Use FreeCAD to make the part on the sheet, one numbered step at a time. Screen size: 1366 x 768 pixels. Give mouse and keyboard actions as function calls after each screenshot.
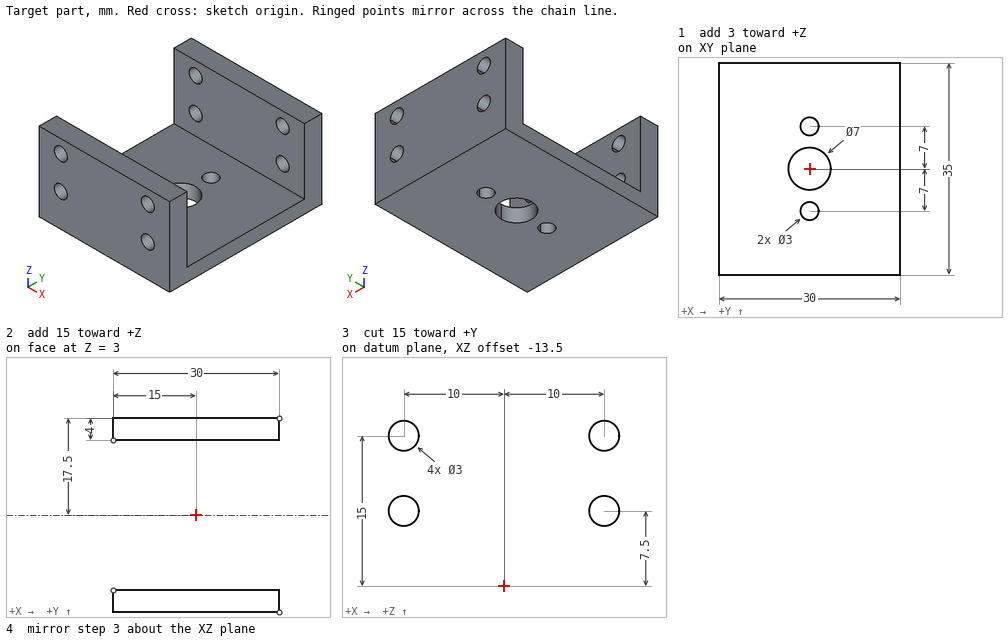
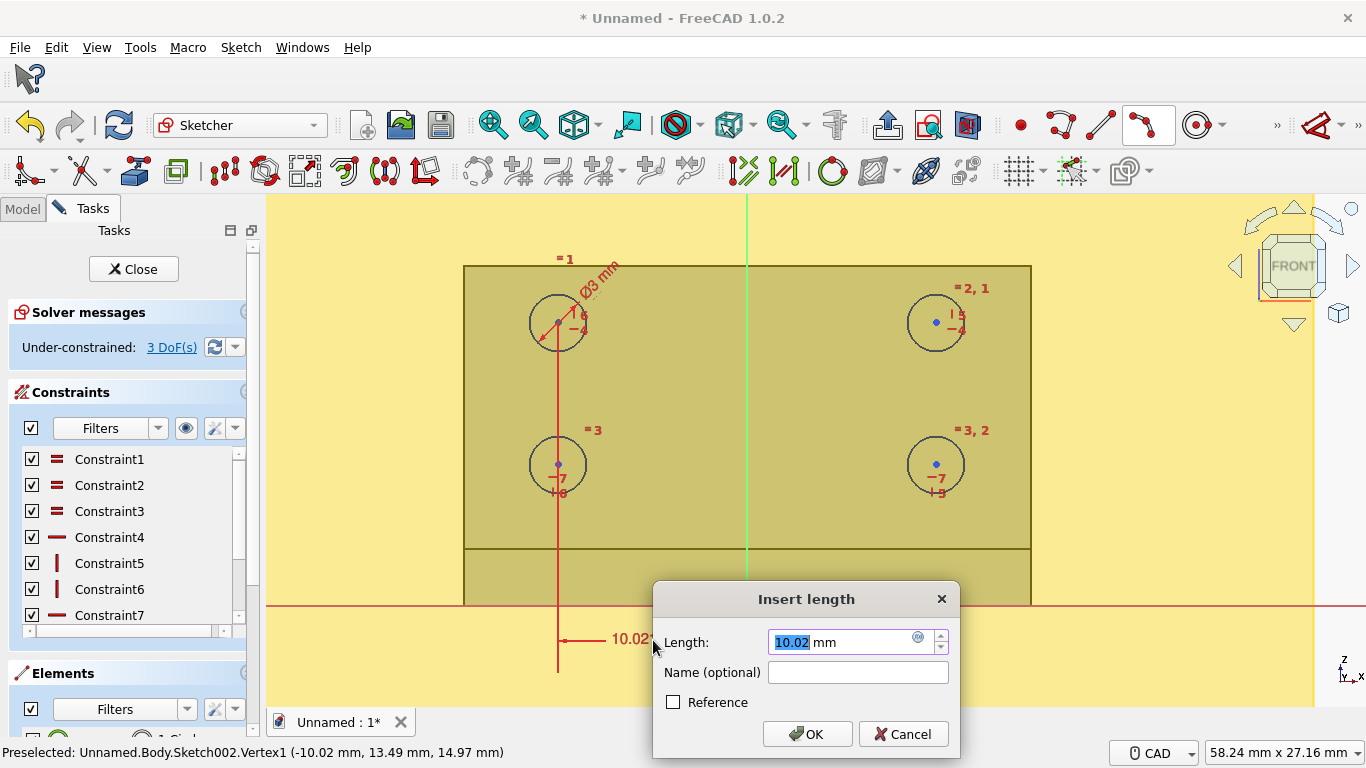
text(10)
key(Return)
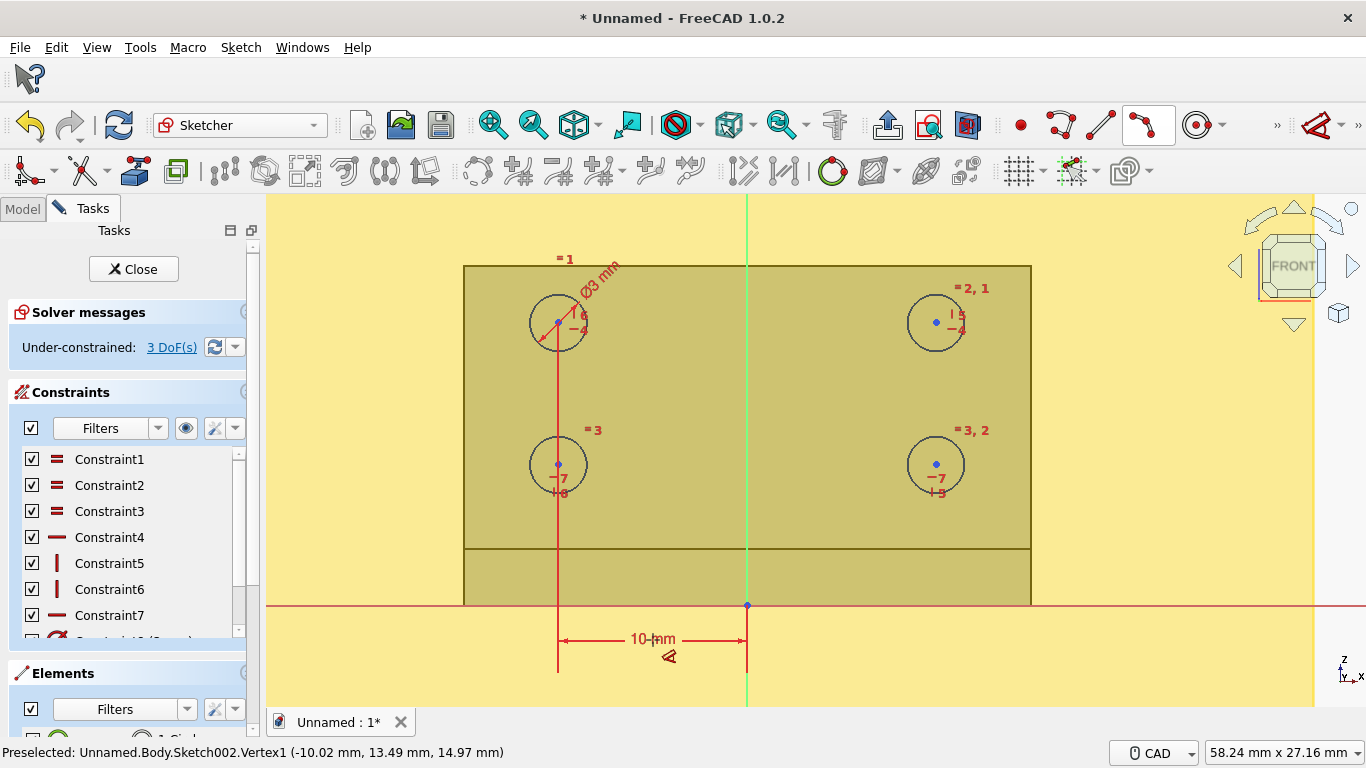
click(558, 323)
click(524, 399)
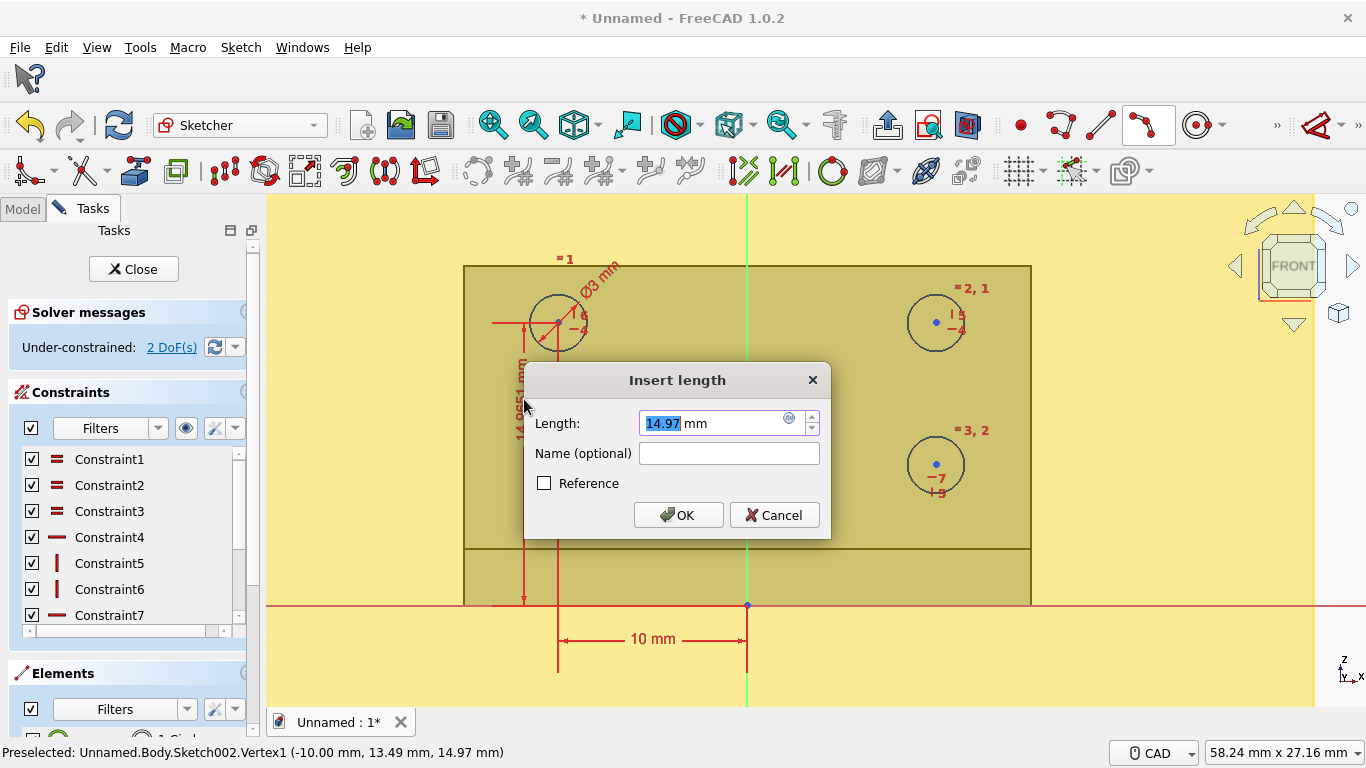
text(15)
key(Return)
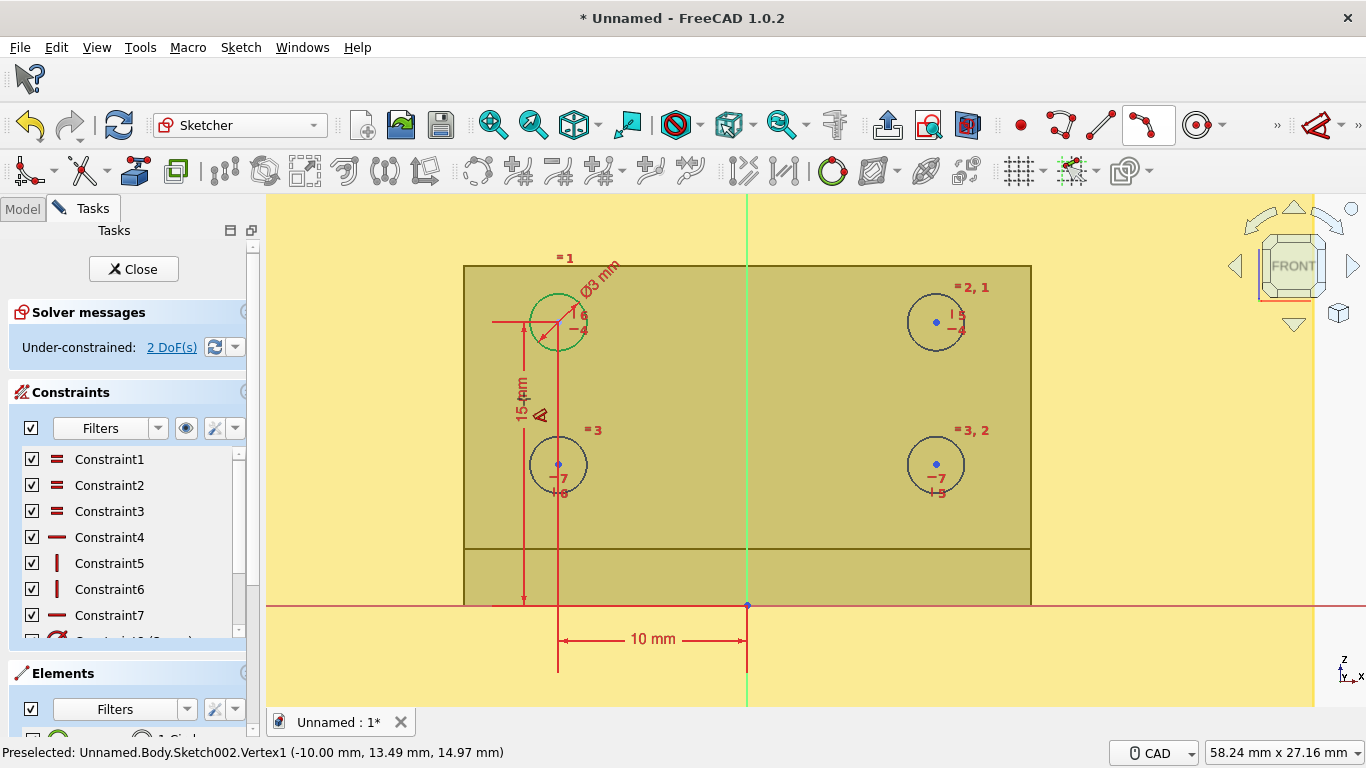
click(936, 322)
click(842, 640)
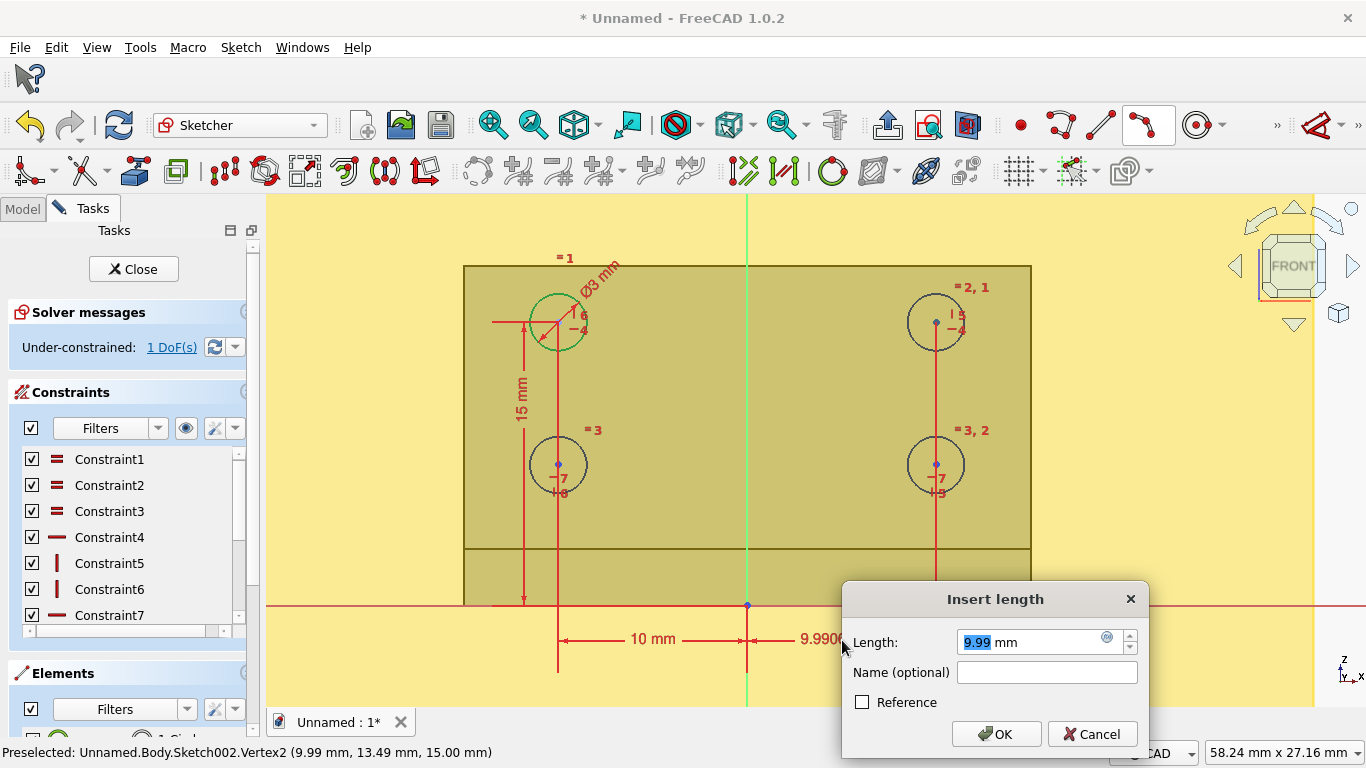
text(10)
key(Return)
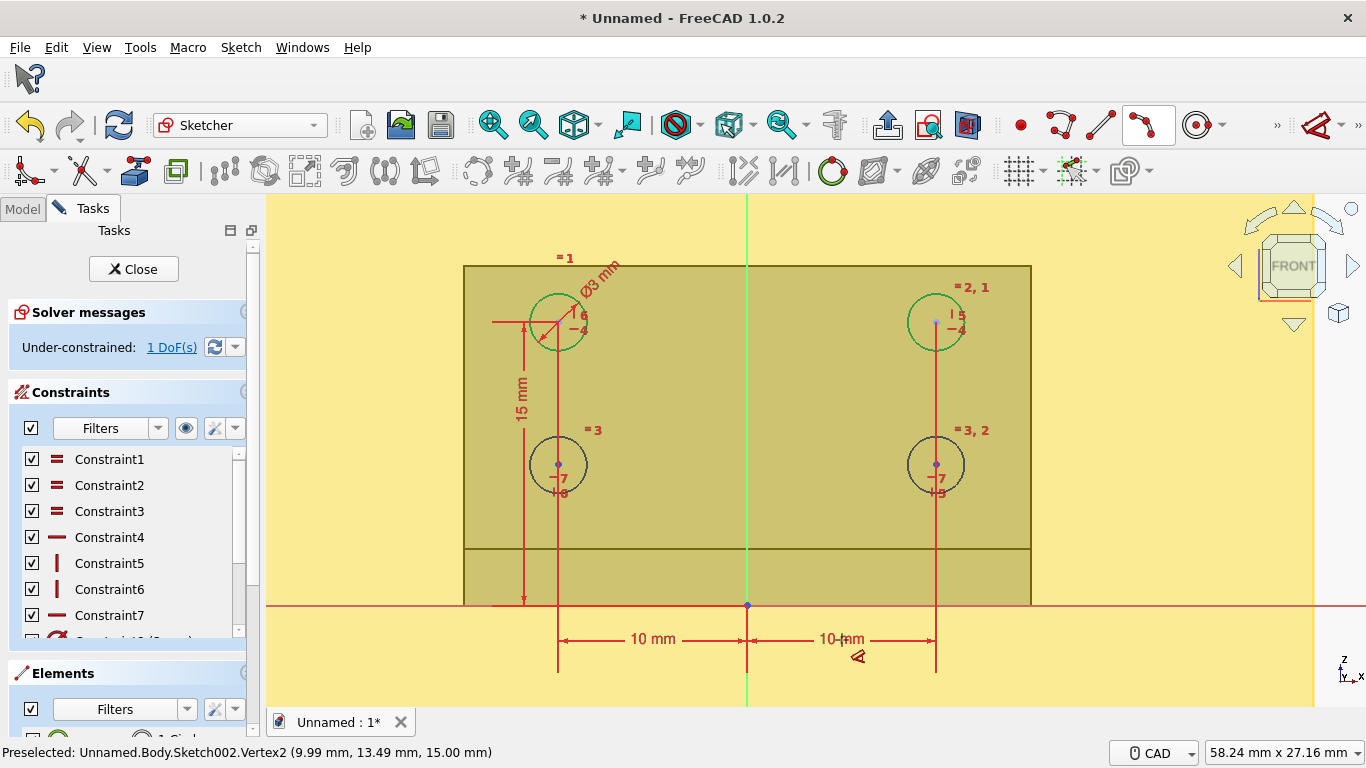
click(936, 465)
click(970, 535)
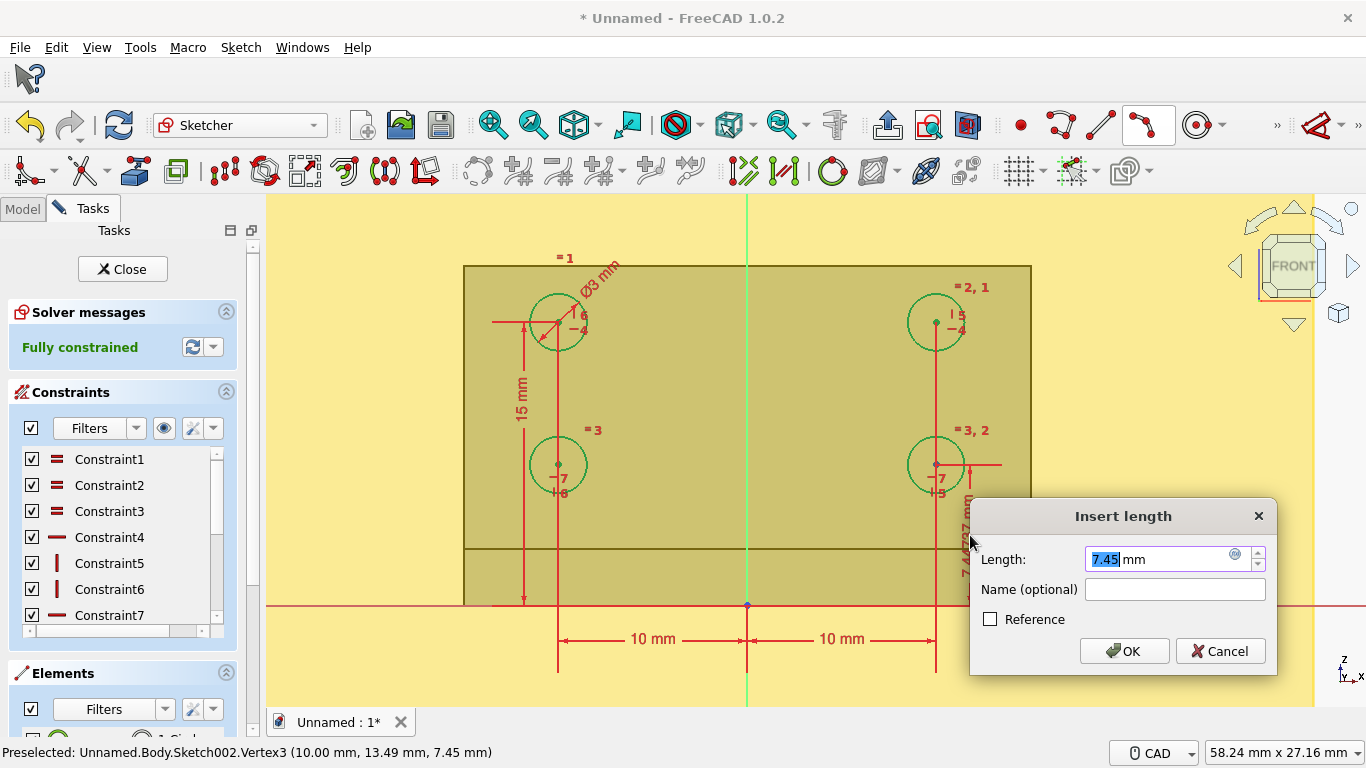
text(7.5)
key(Return)
key(Escape)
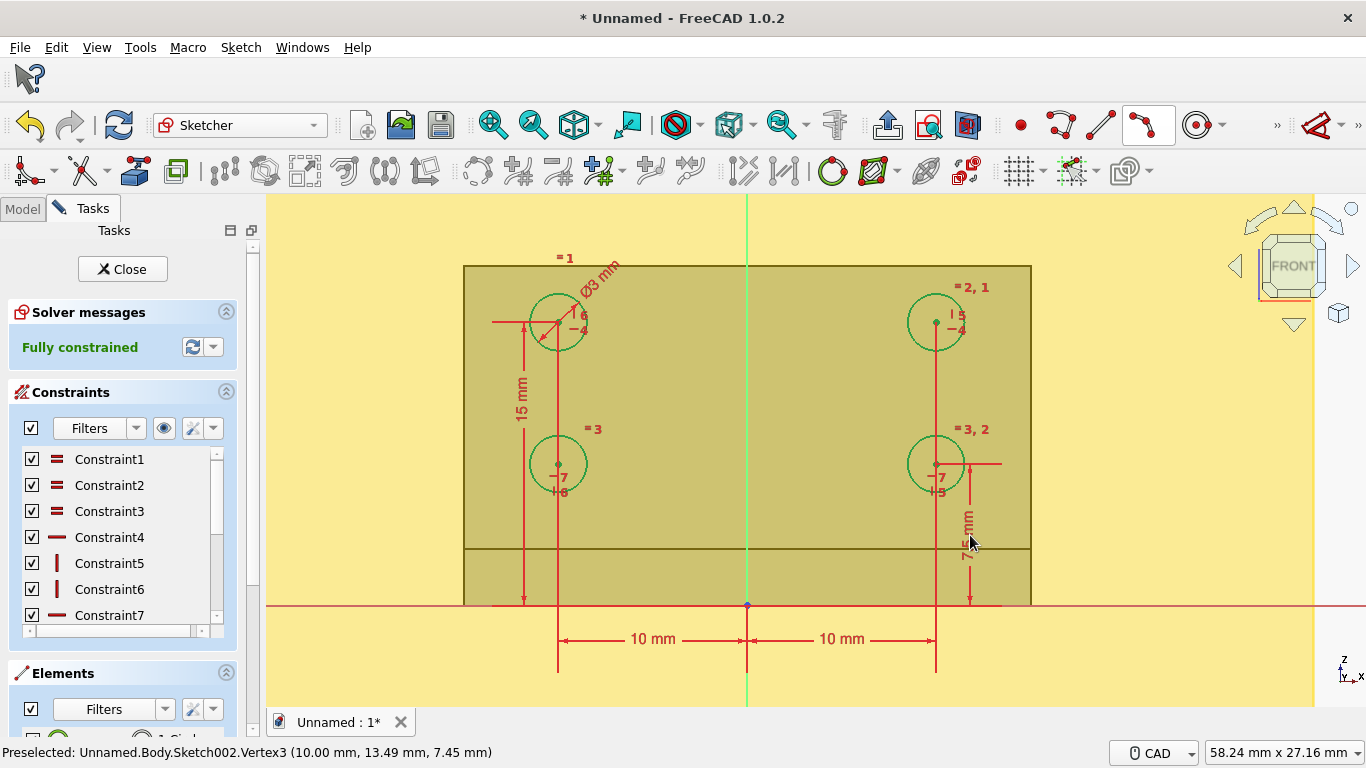
click(123, 269)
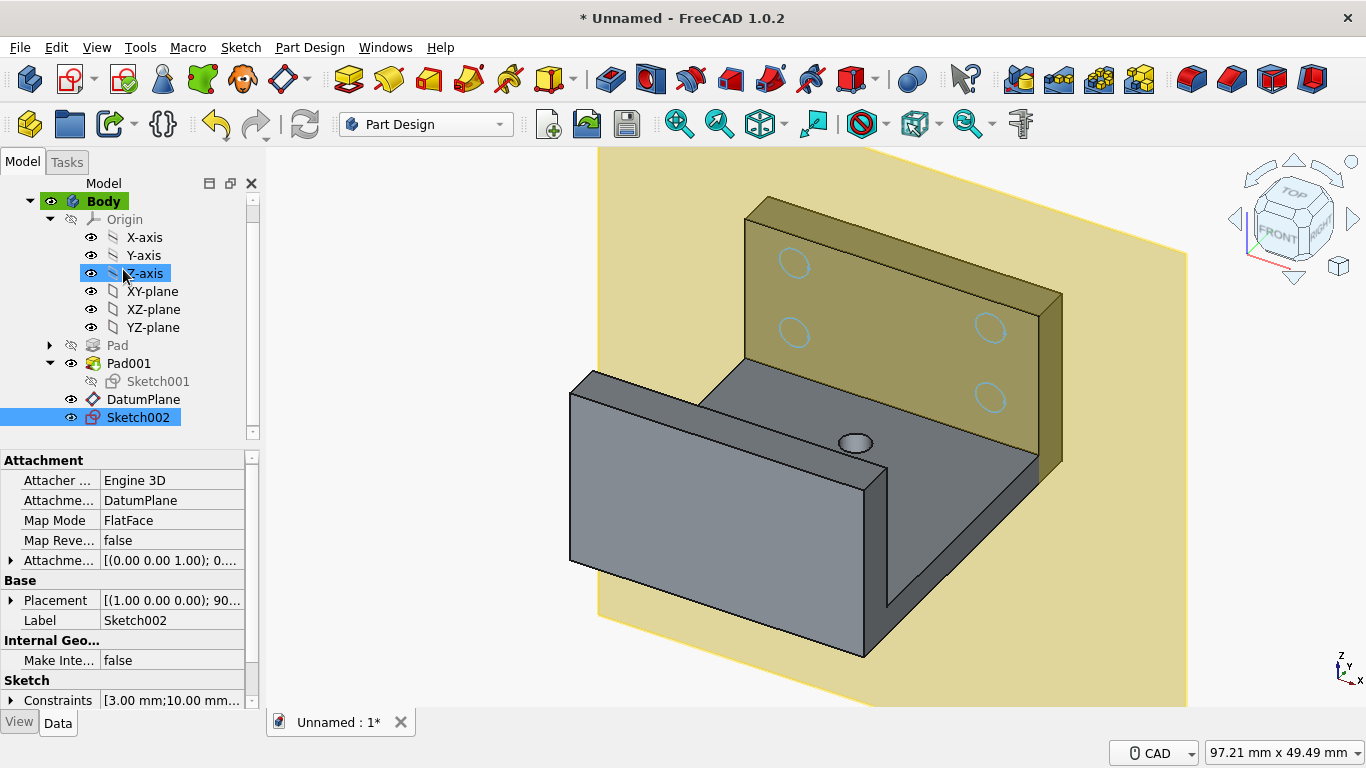
click(612, 80)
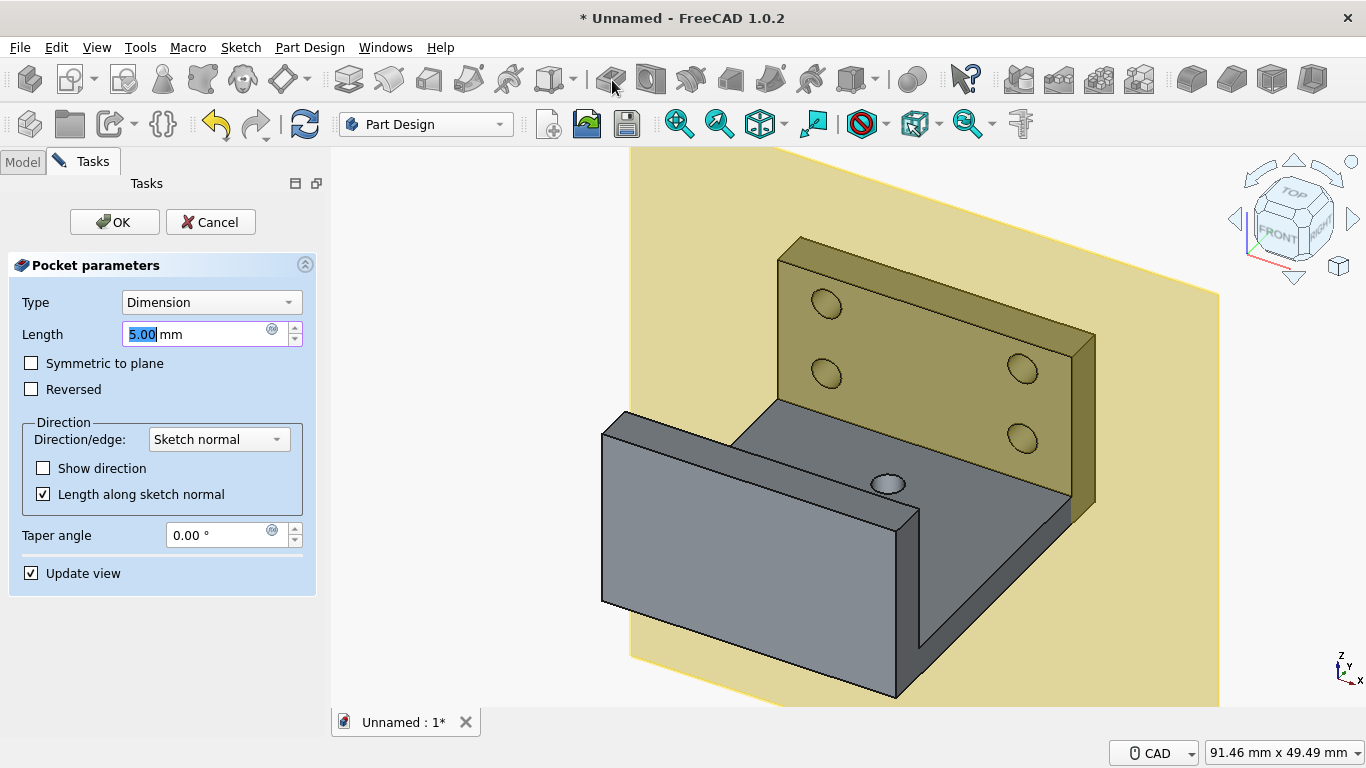
text(15)
key(Tab)